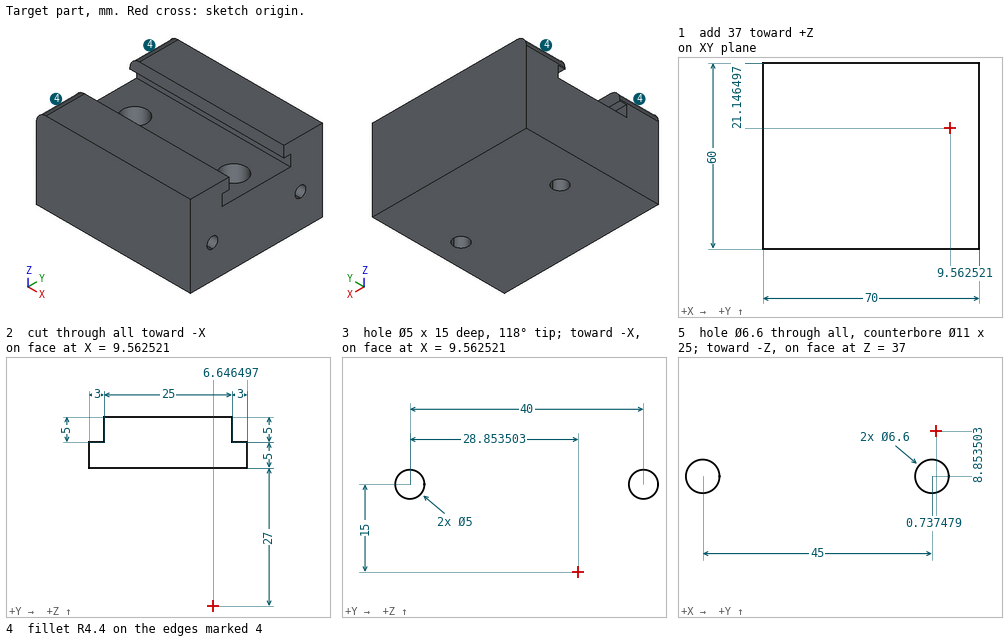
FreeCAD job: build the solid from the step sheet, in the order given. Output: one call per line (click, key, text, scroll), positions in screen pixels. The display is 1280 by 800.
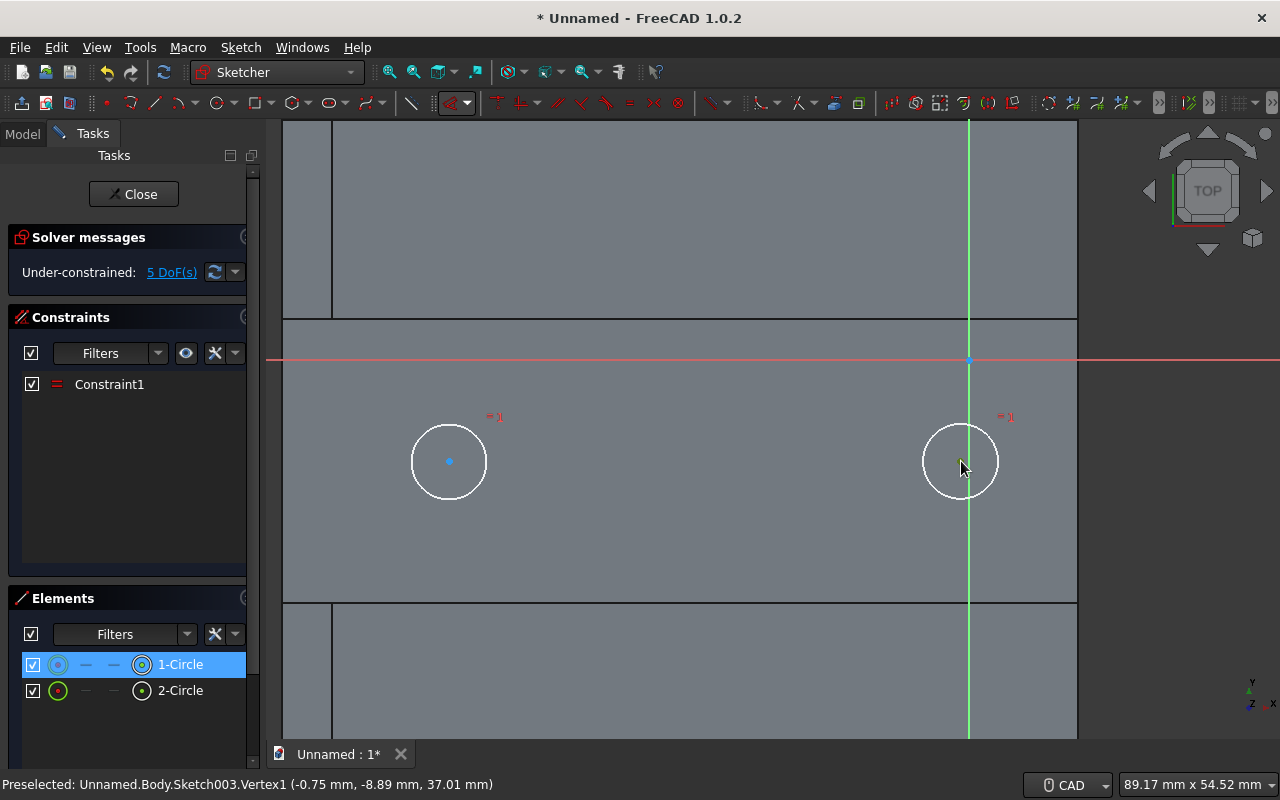
click(449, 462)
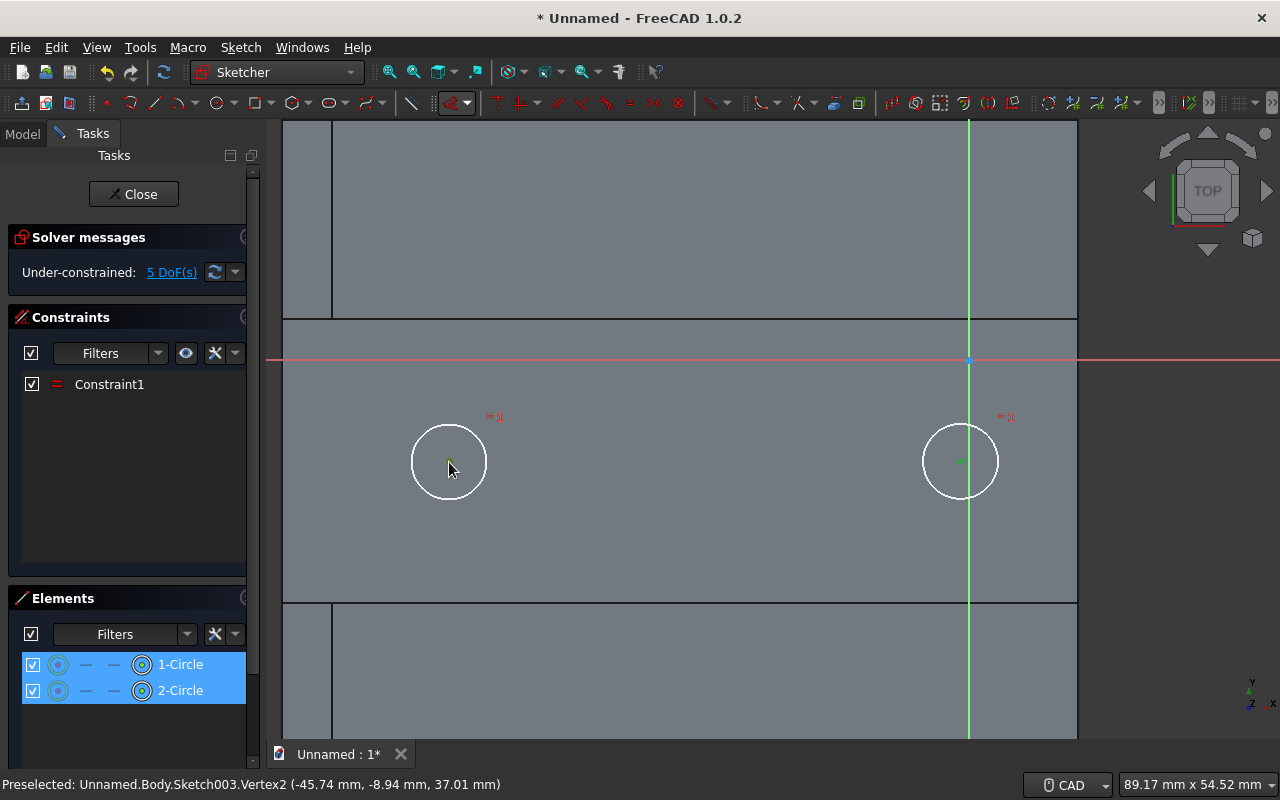
click(540, 104)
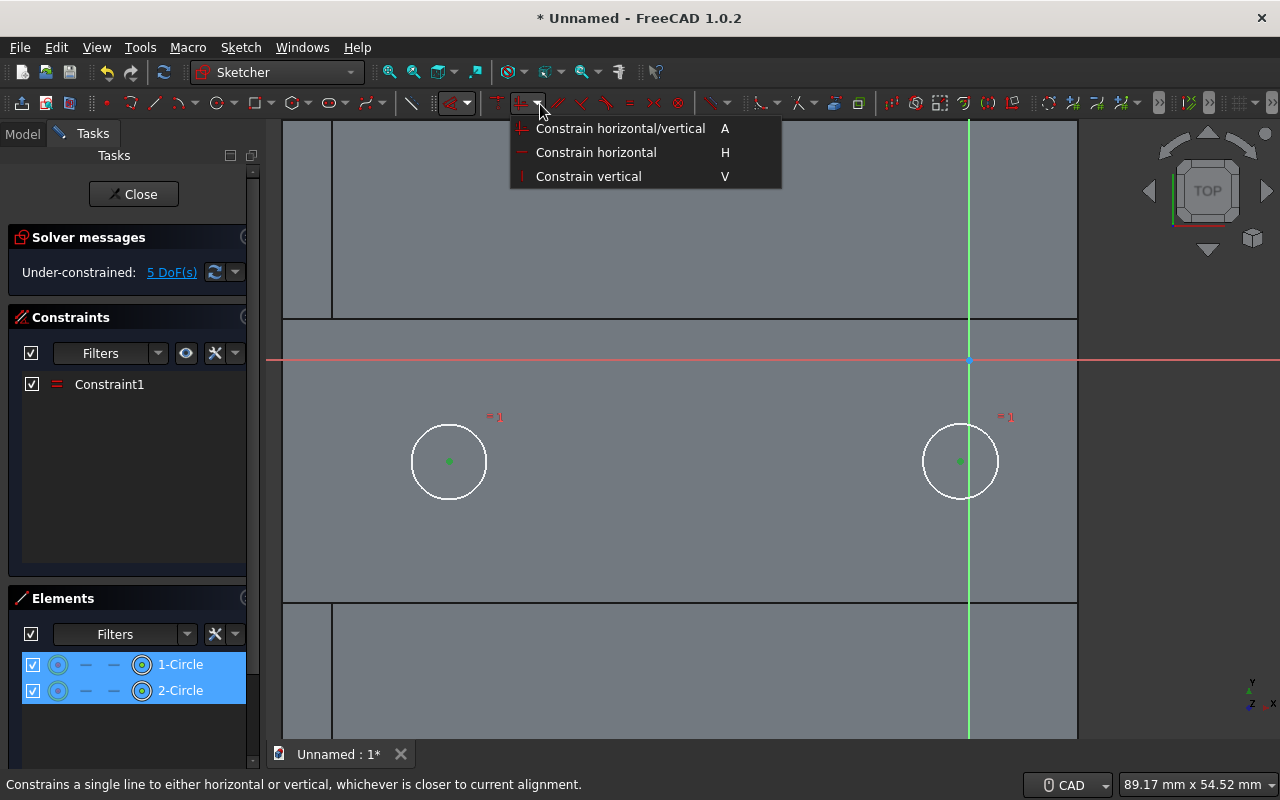
click(646, 152)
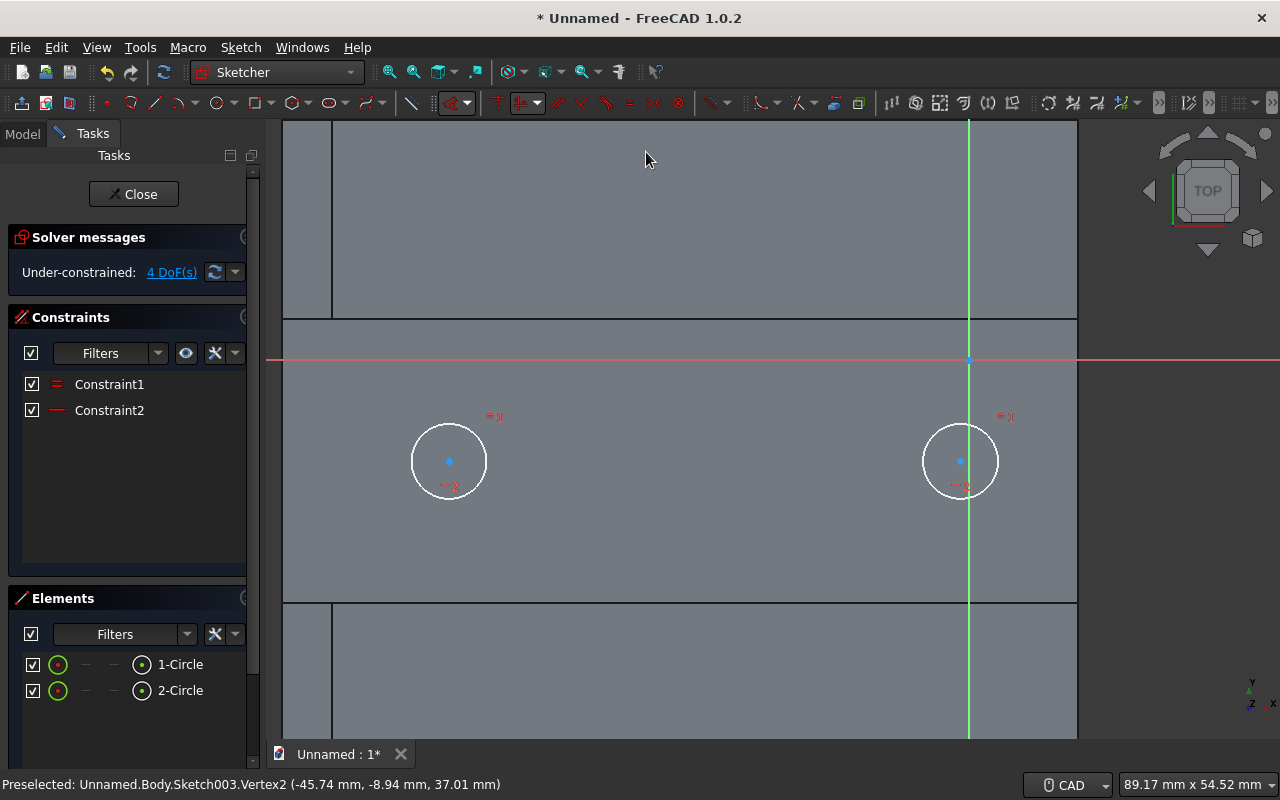
click(987, 435)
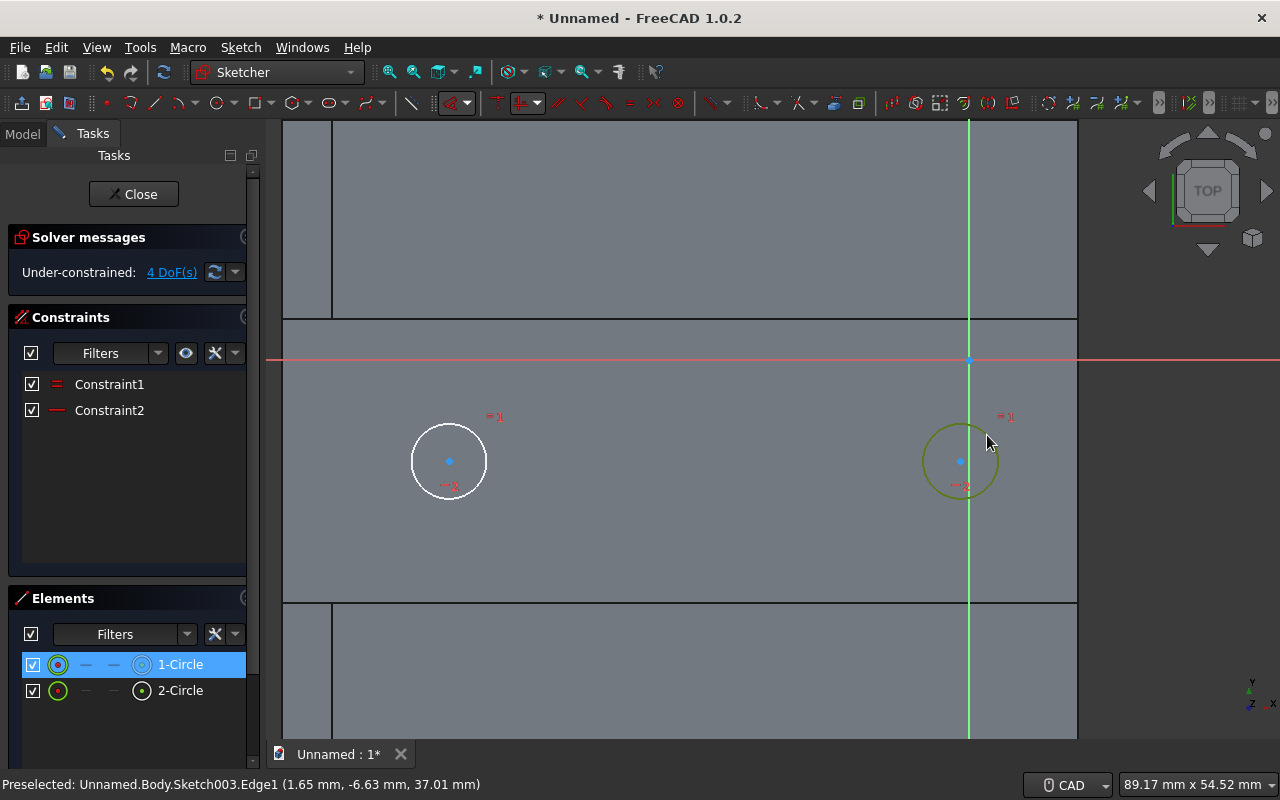
key(k)
key(o)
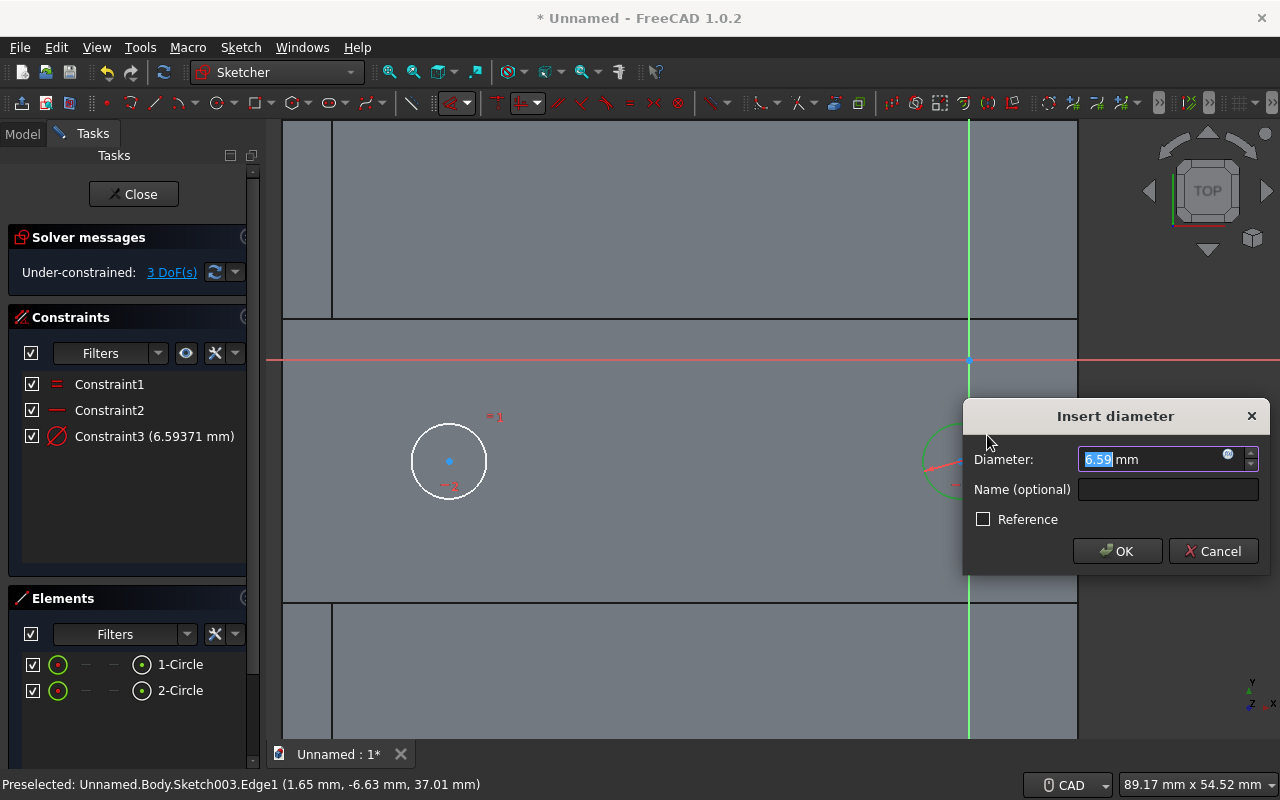
text(6.6)
key(Return)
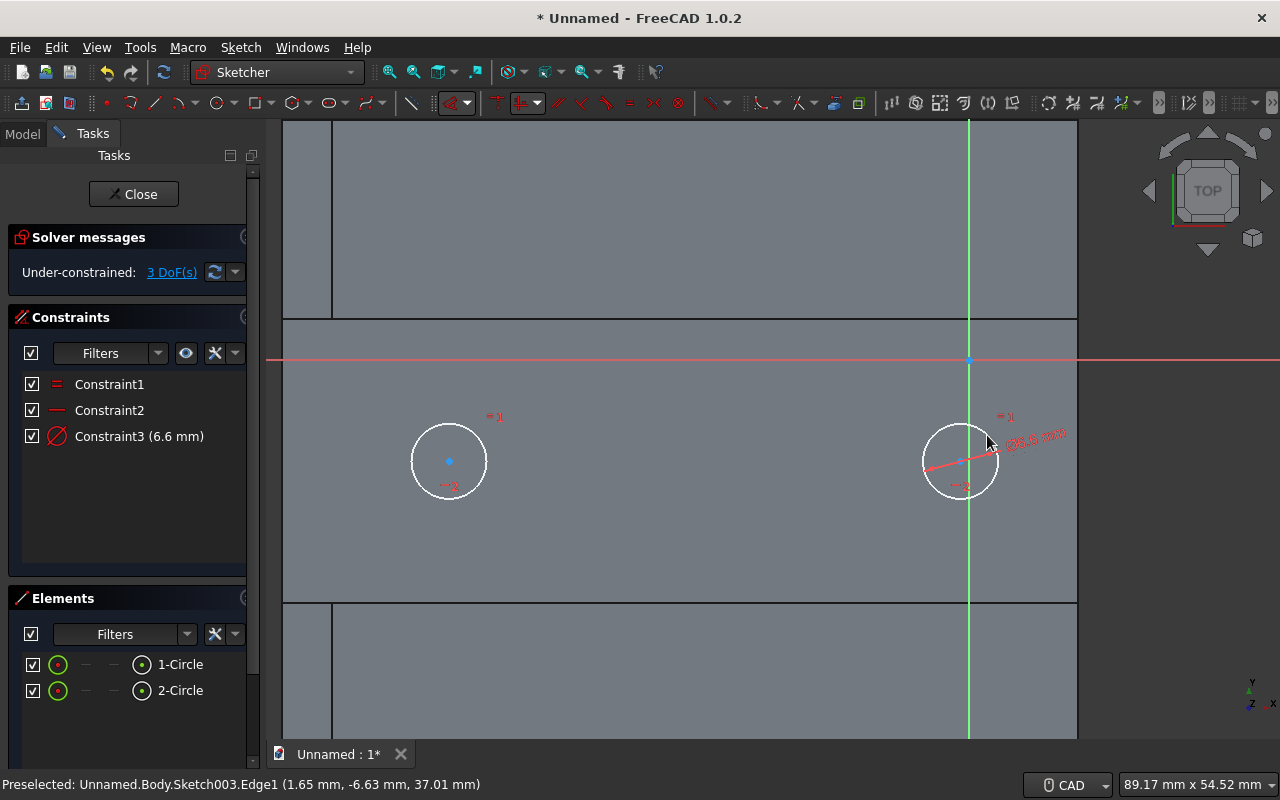
click(961, 461)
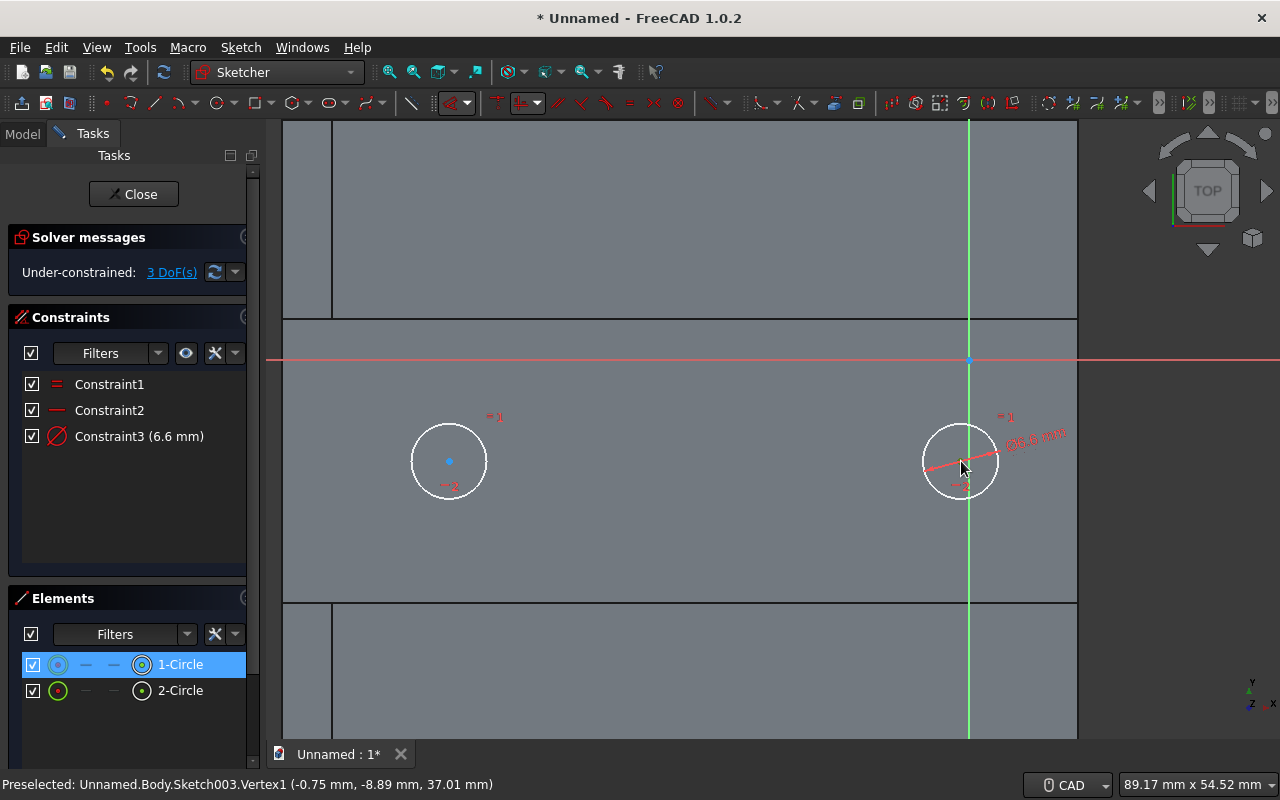
click(449, 461)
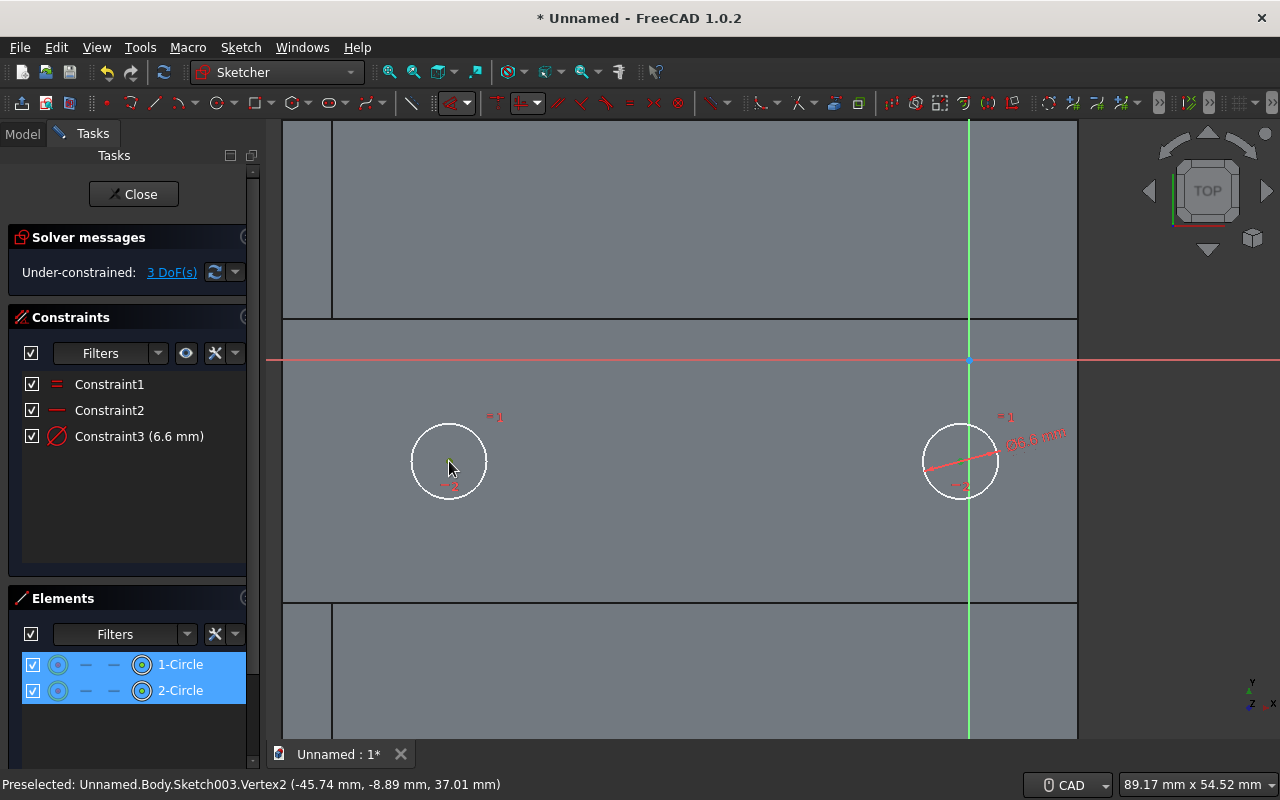
click(470, 104)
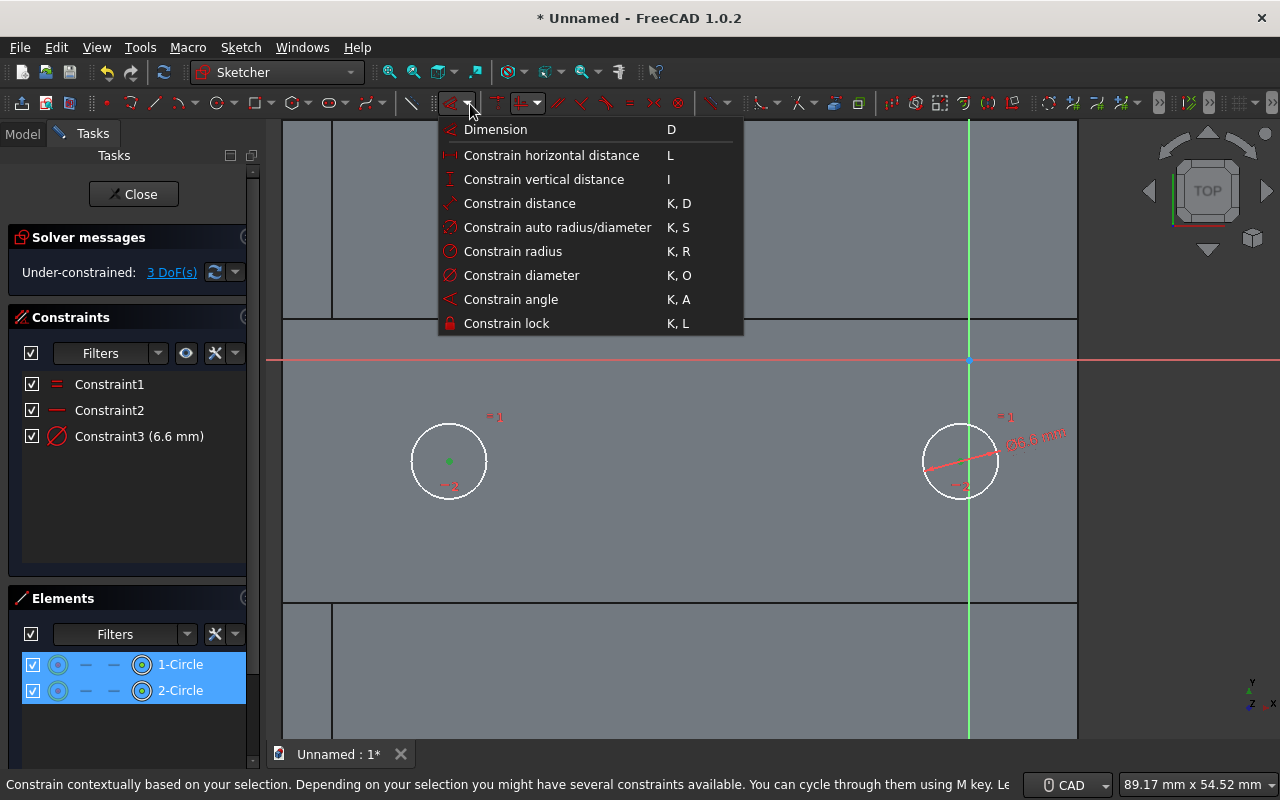
click(591, 155)